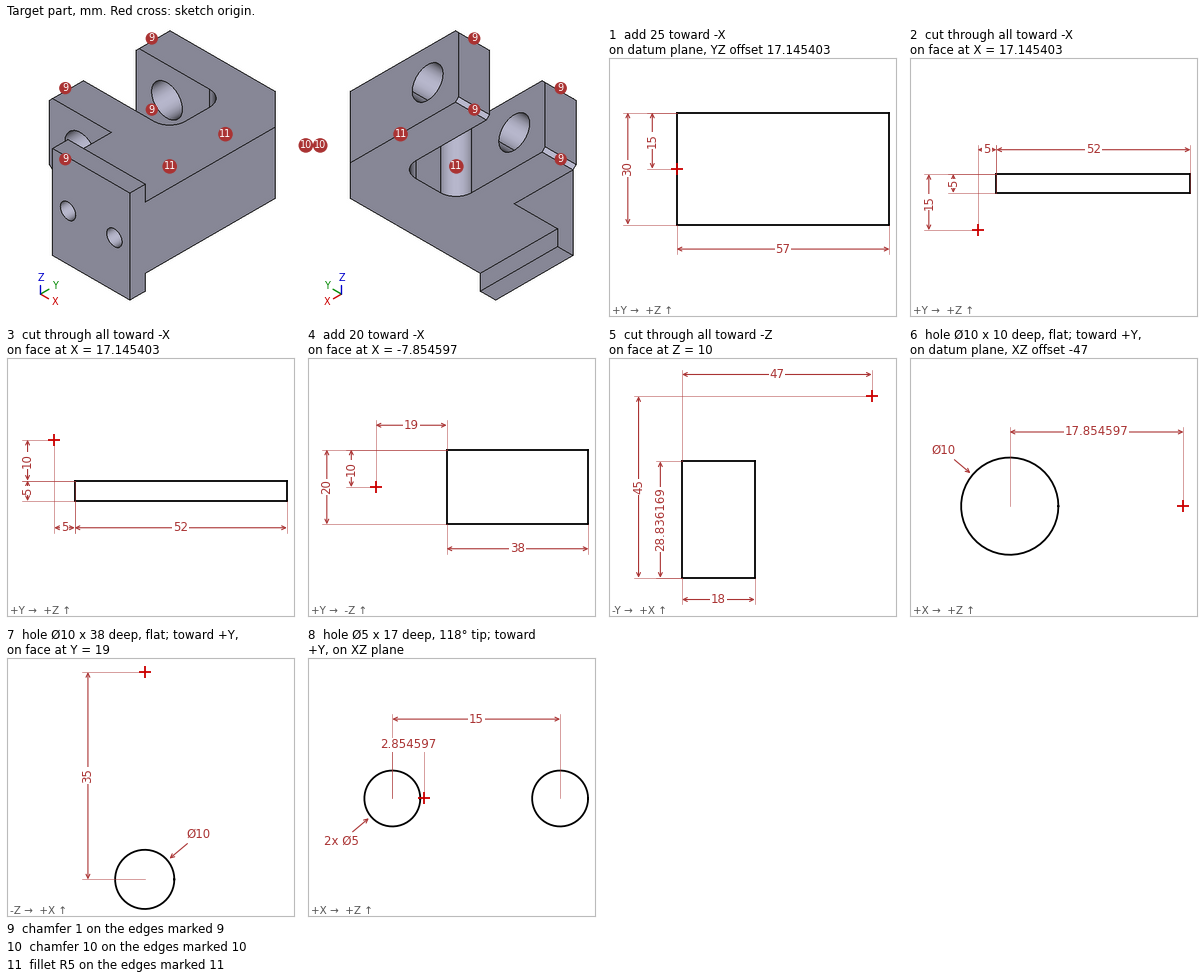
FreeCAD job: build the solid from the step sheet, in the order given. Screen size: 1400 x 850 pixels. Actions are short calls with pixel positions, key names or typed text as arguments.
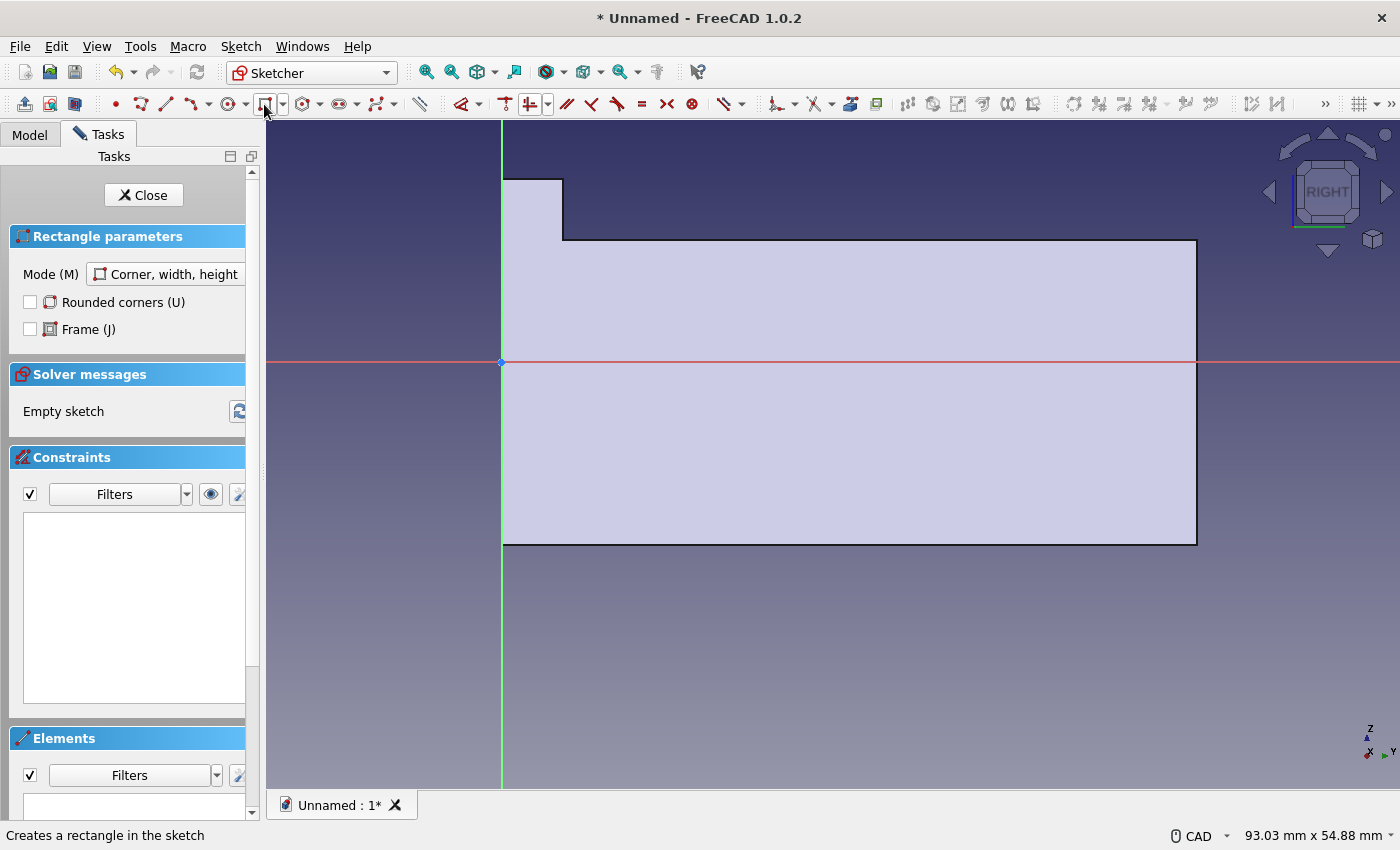
click(563, 484)
click(1197, 545)
key(Escape)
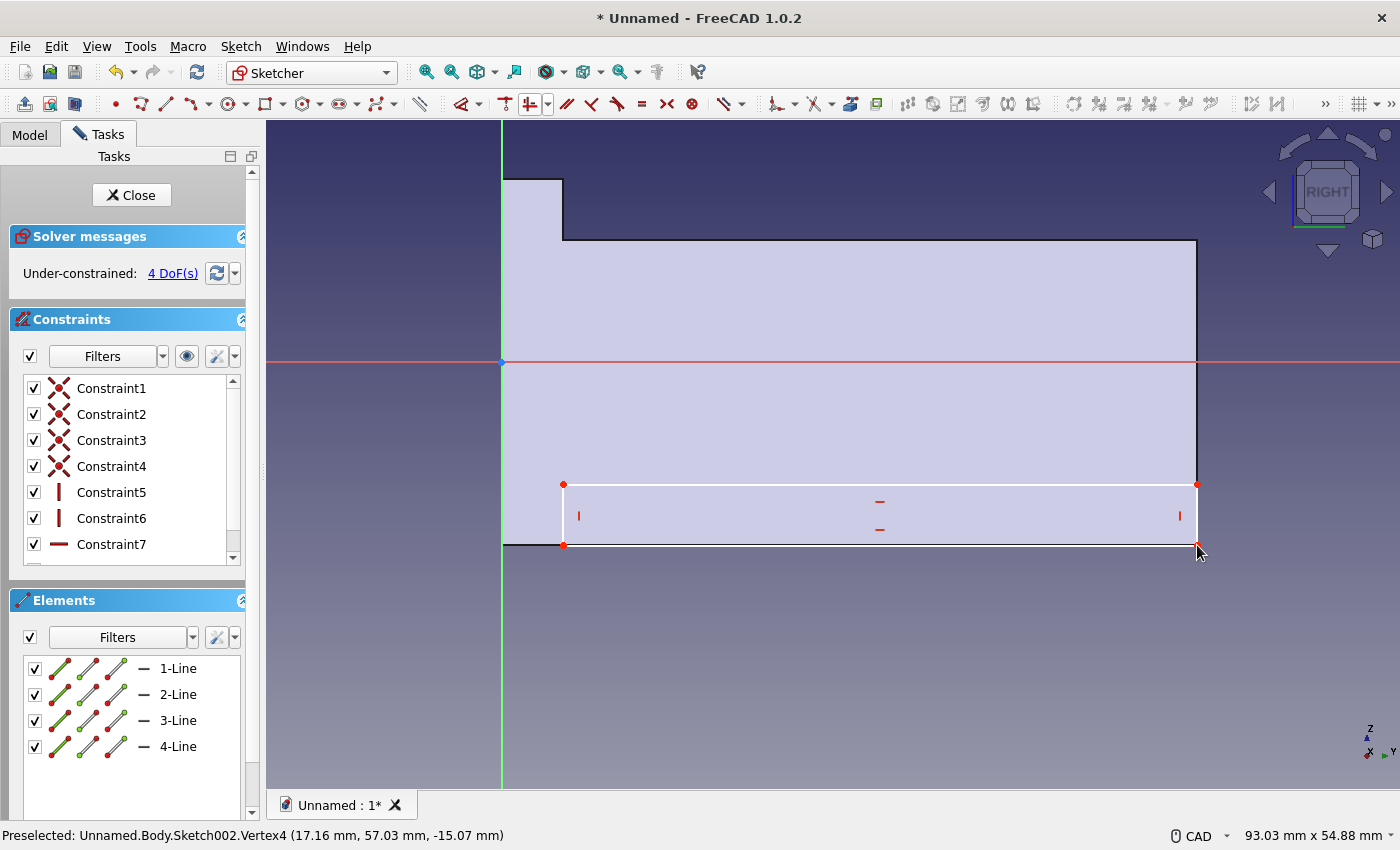
click(460, 104)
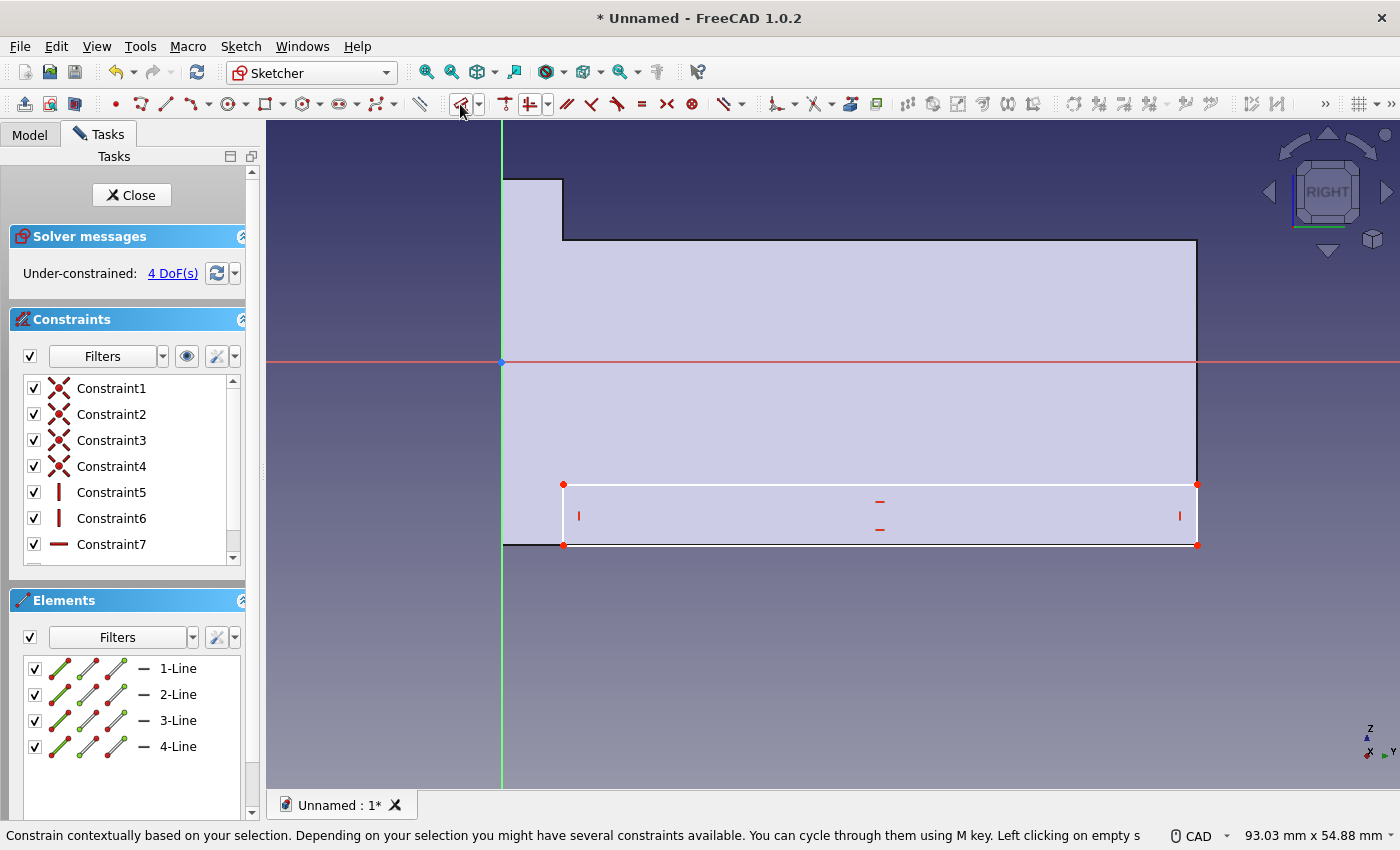
click(563, 503)
click(529, 515)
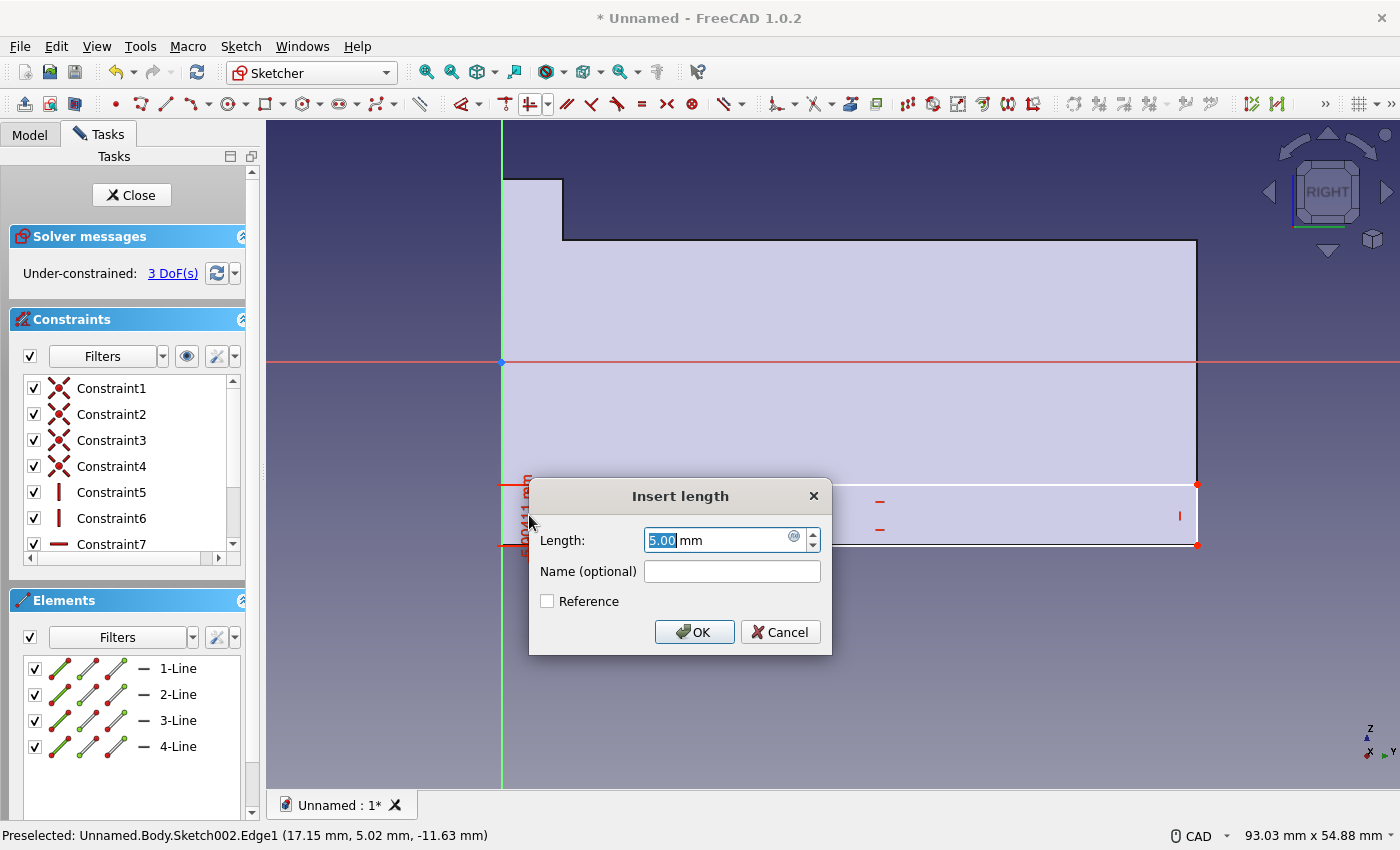
text(5)
key(Return)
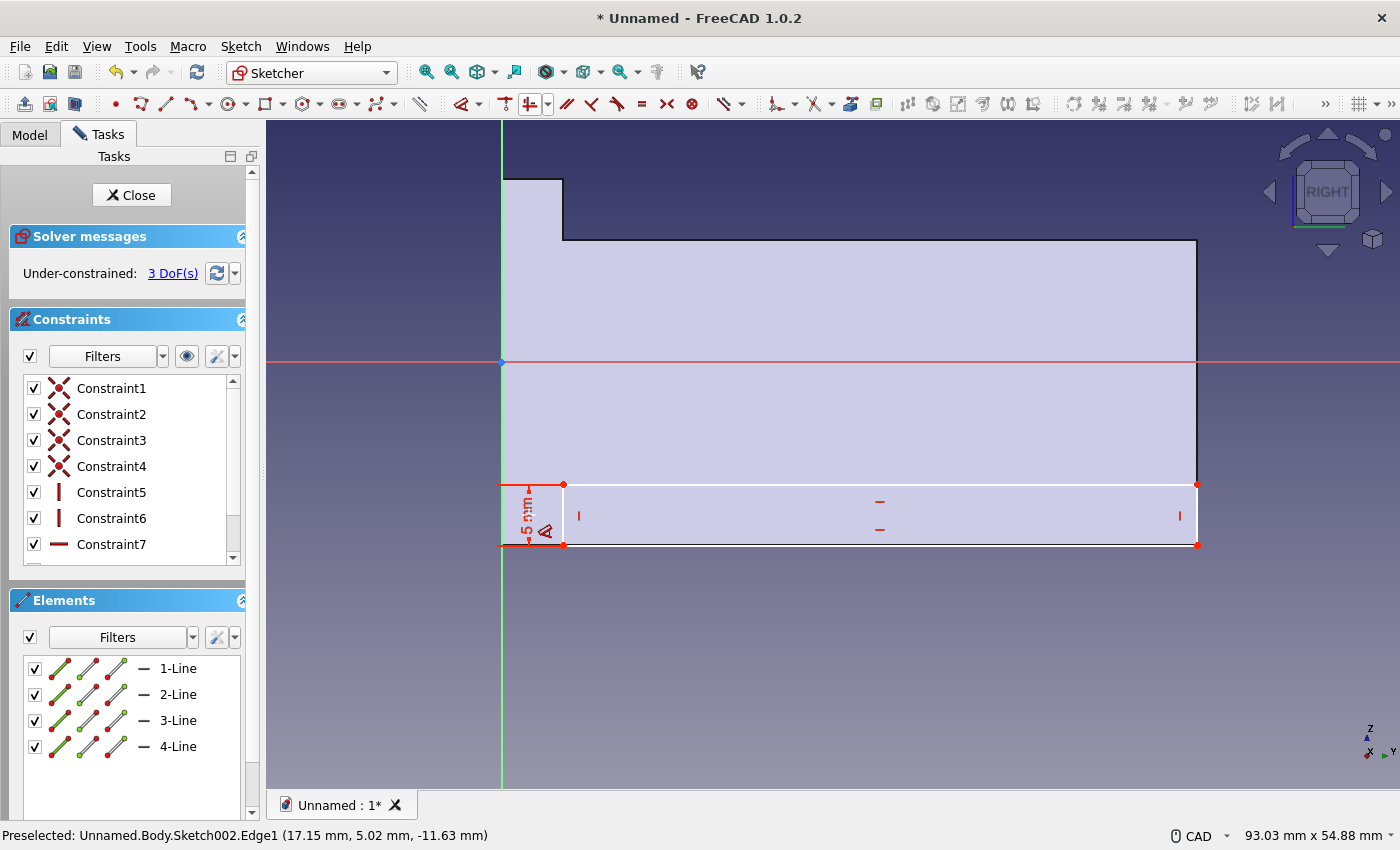
click(753, 546)
click(880, 580)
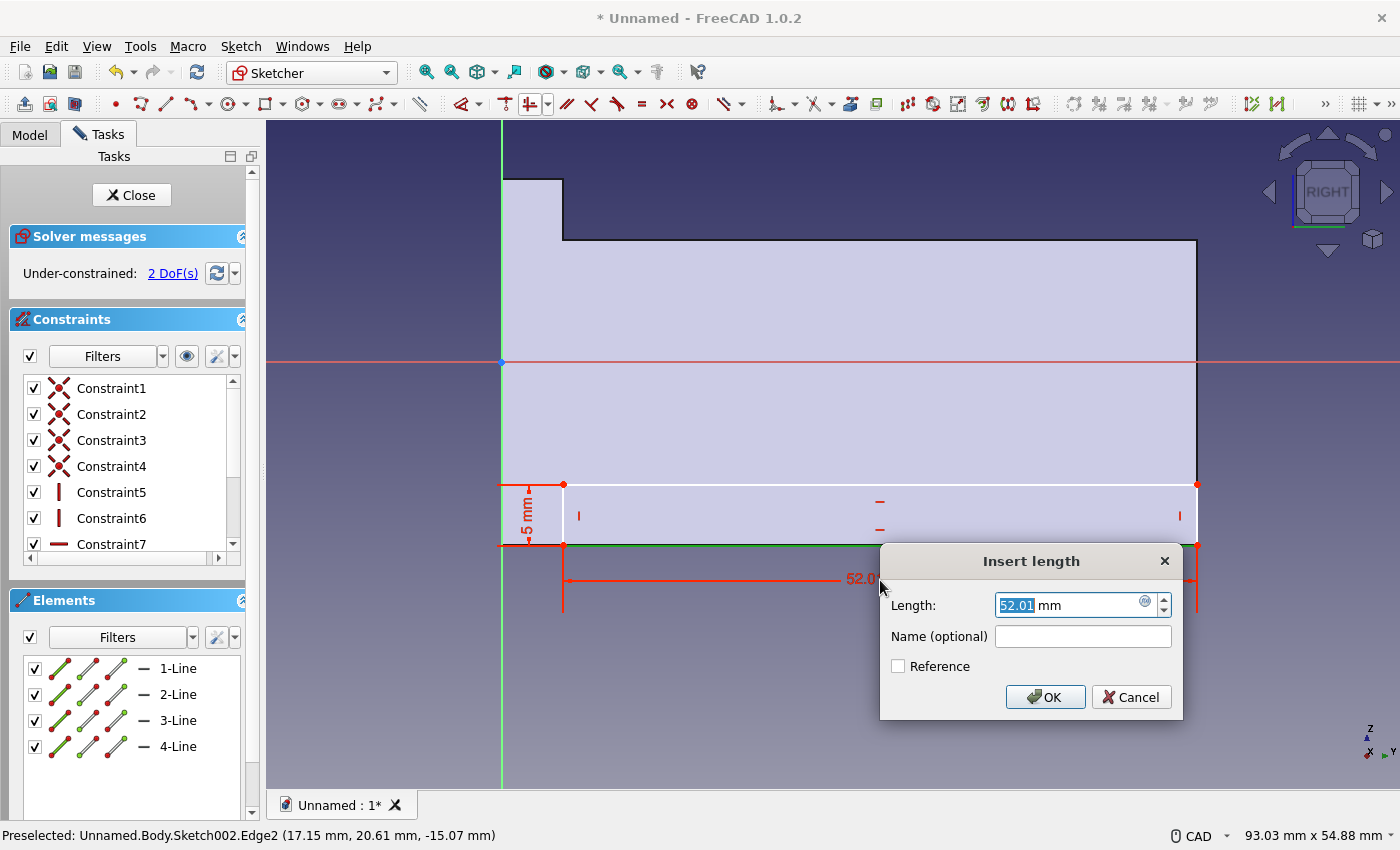
text(52)
key(Return)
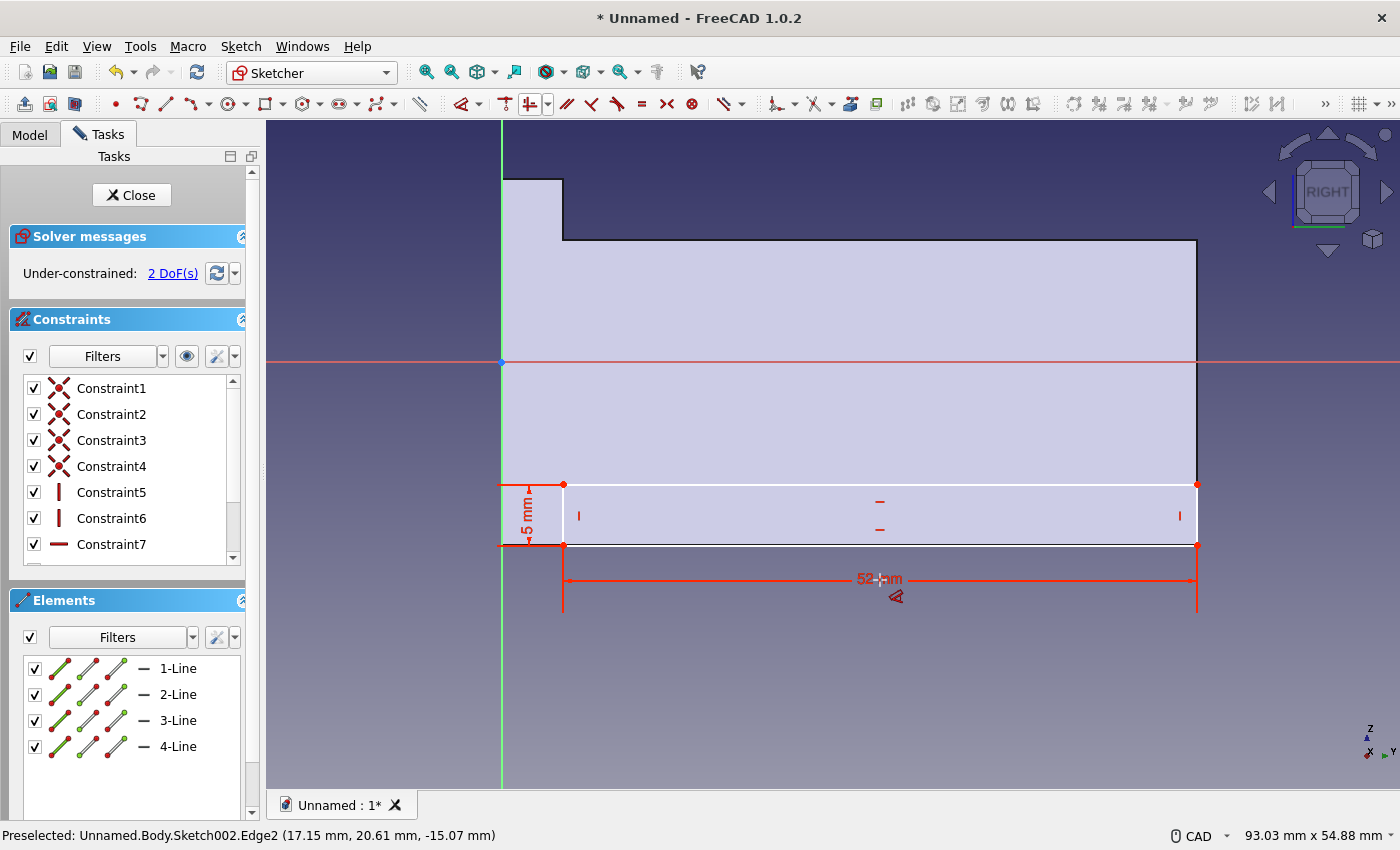
click(563, 485)
click(532, 328)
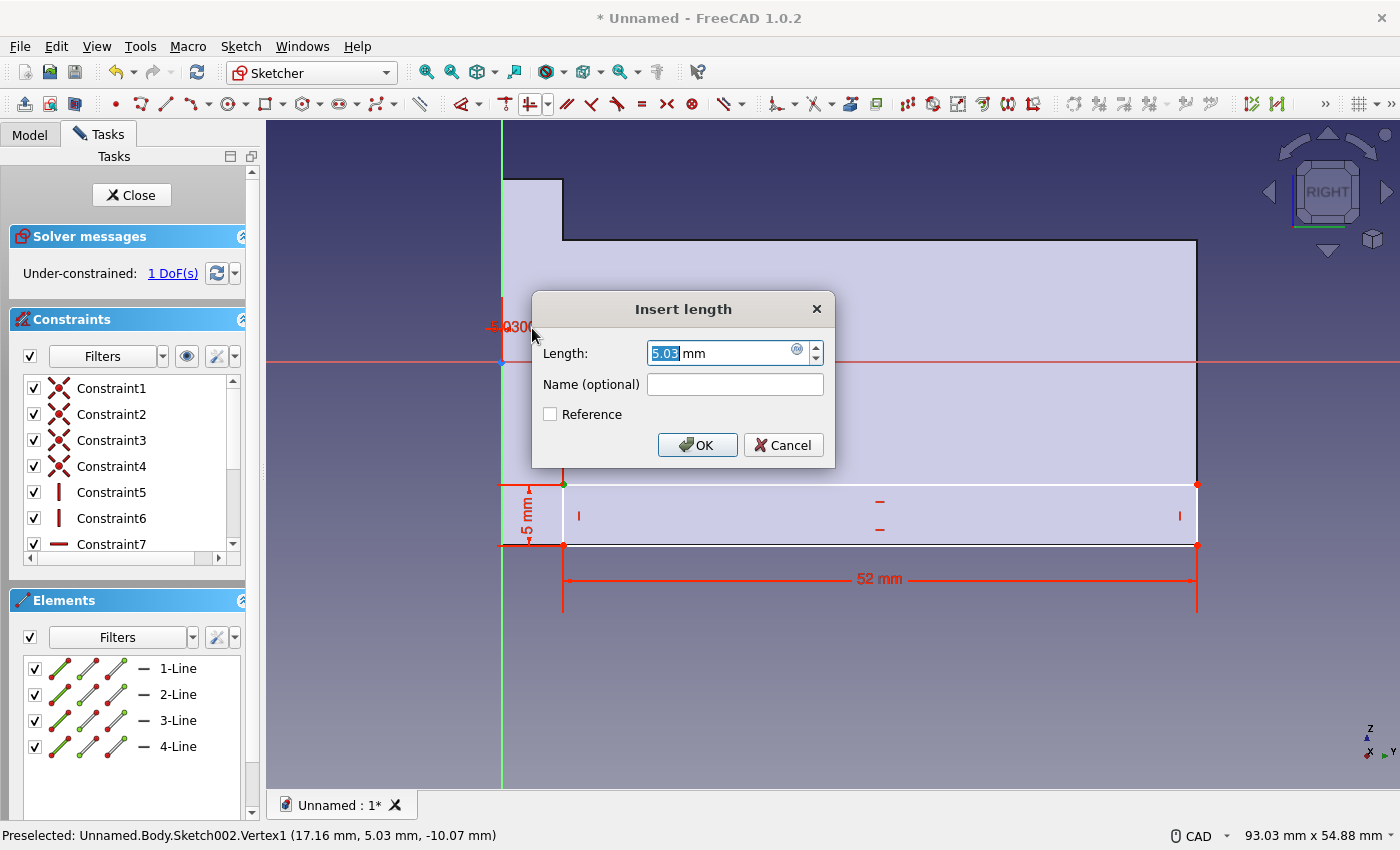
text(5)
key(Return)